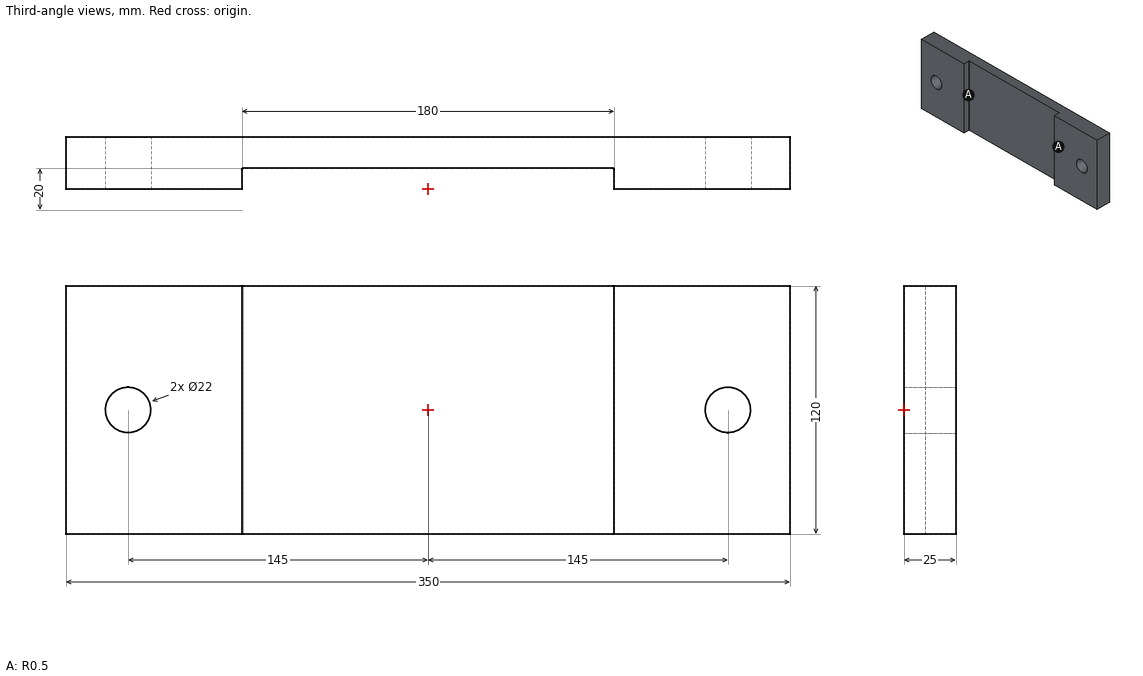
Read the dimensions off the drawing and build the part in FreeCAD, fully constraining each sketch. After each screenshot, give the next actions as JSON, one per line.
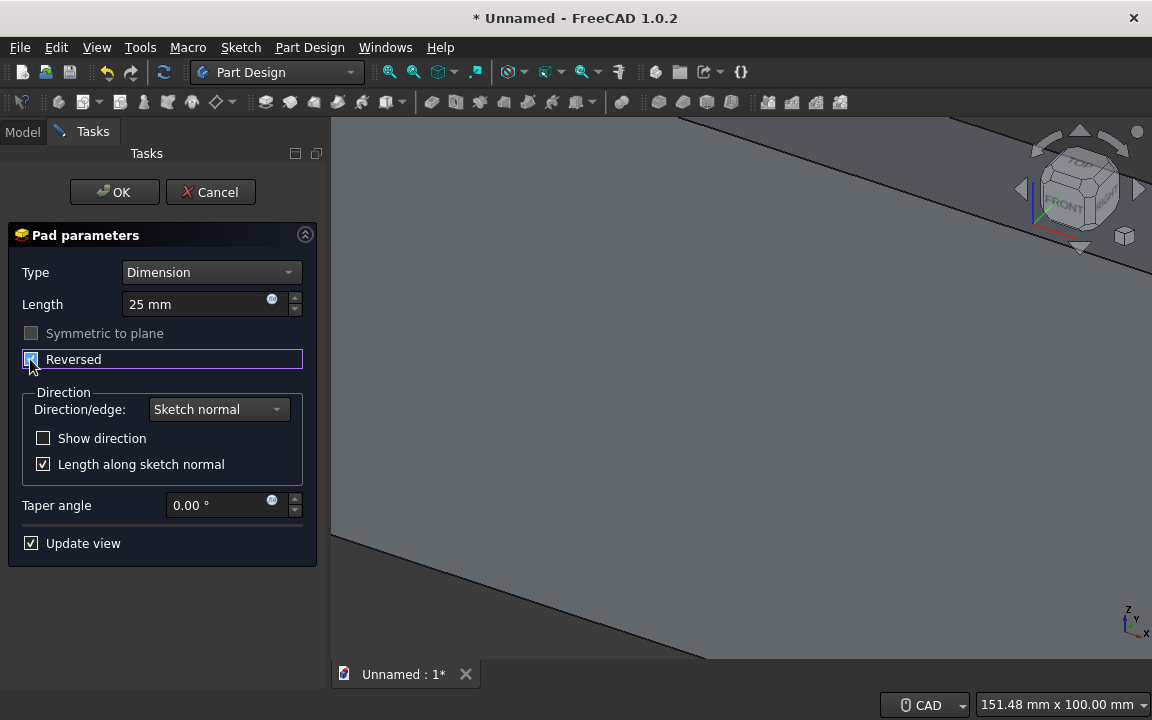
{"action": "left_click", "coordinate": [115, 192]}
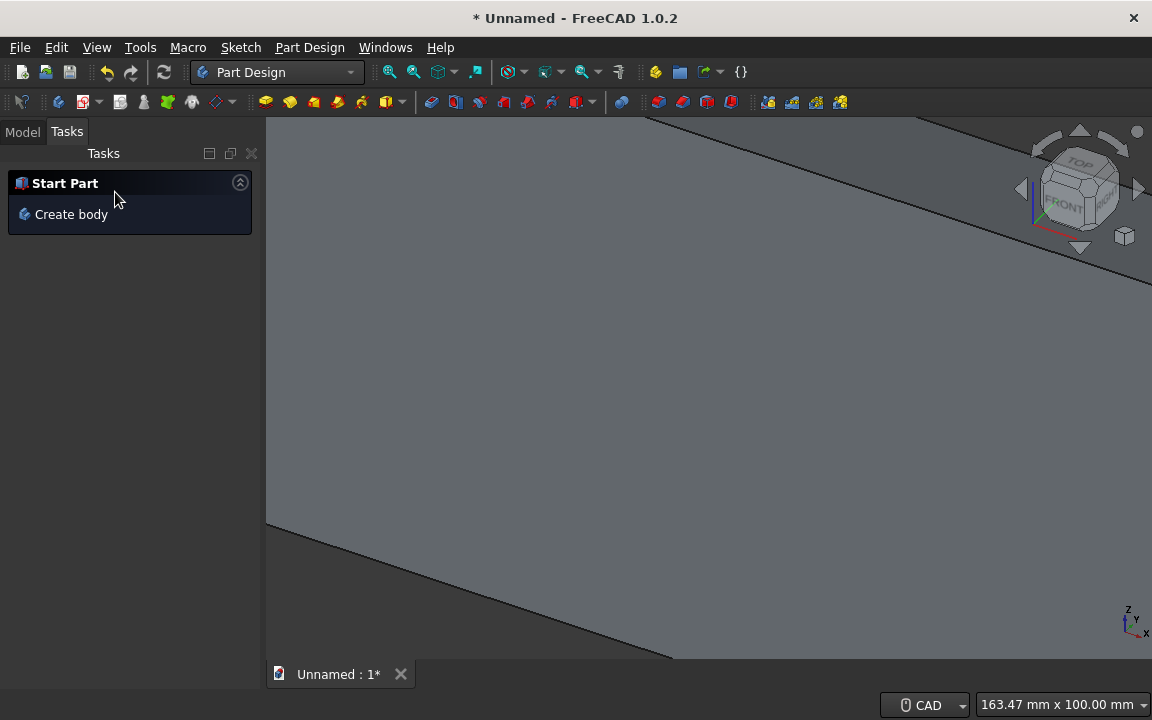
{"action": "left_click", "coordinate": [390, 72]}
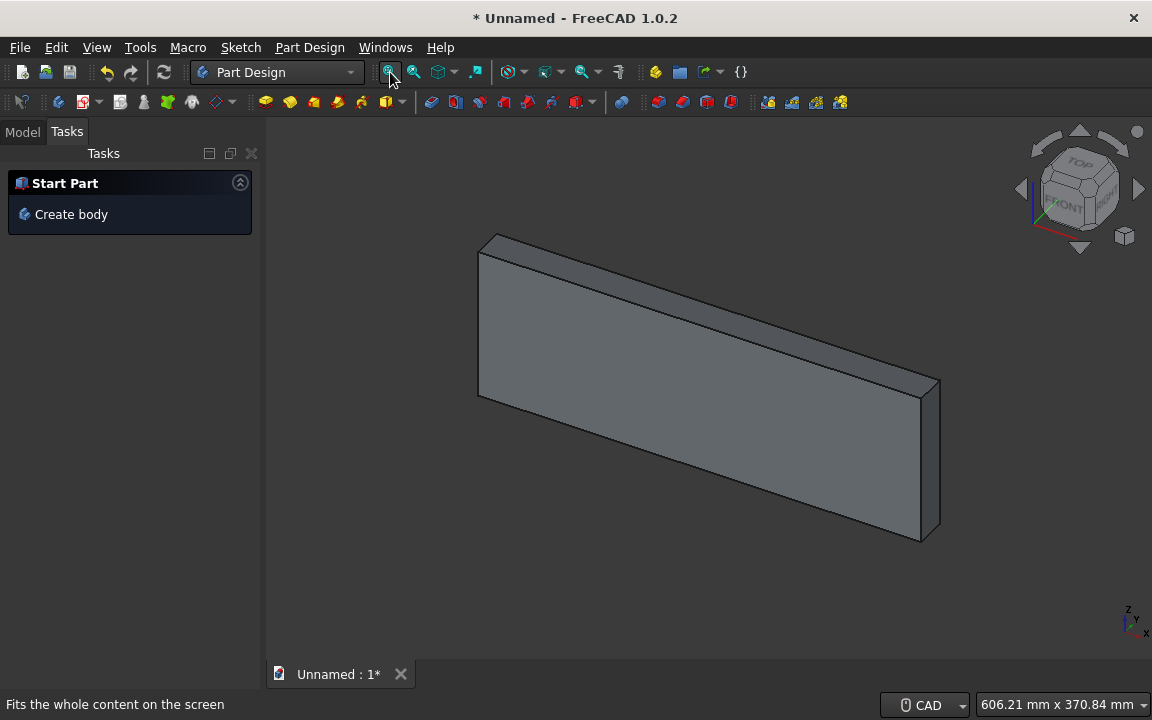
{"action": "left_click", "coordinate": [899, 378]}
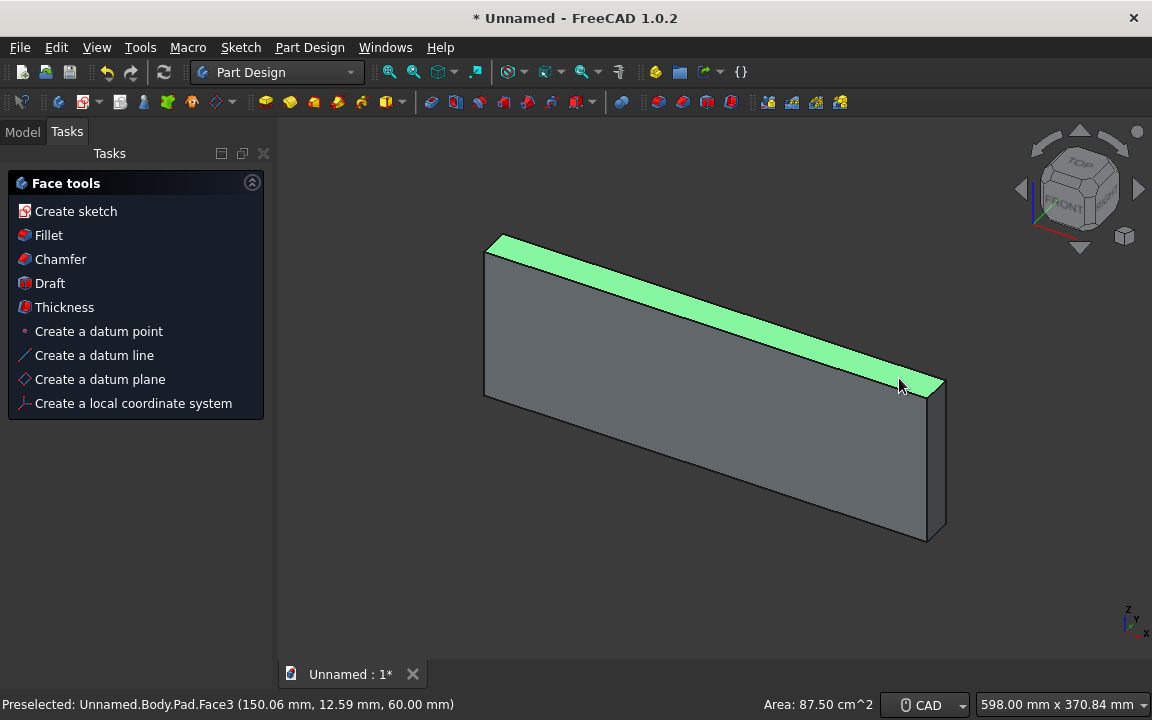
{"action": "left_click", "coordinate": [84, 102]}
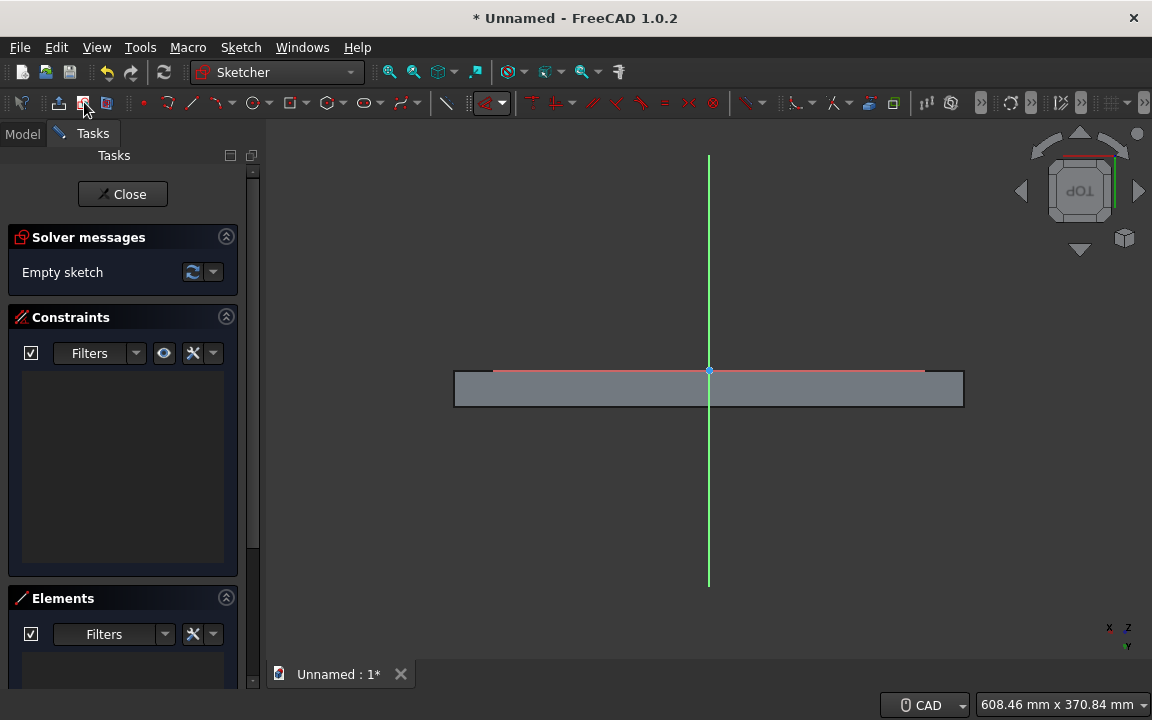
{"action": "scroll", "coordinate": [792, 349], "scroll_direction": "up", "scroll_amount": 3}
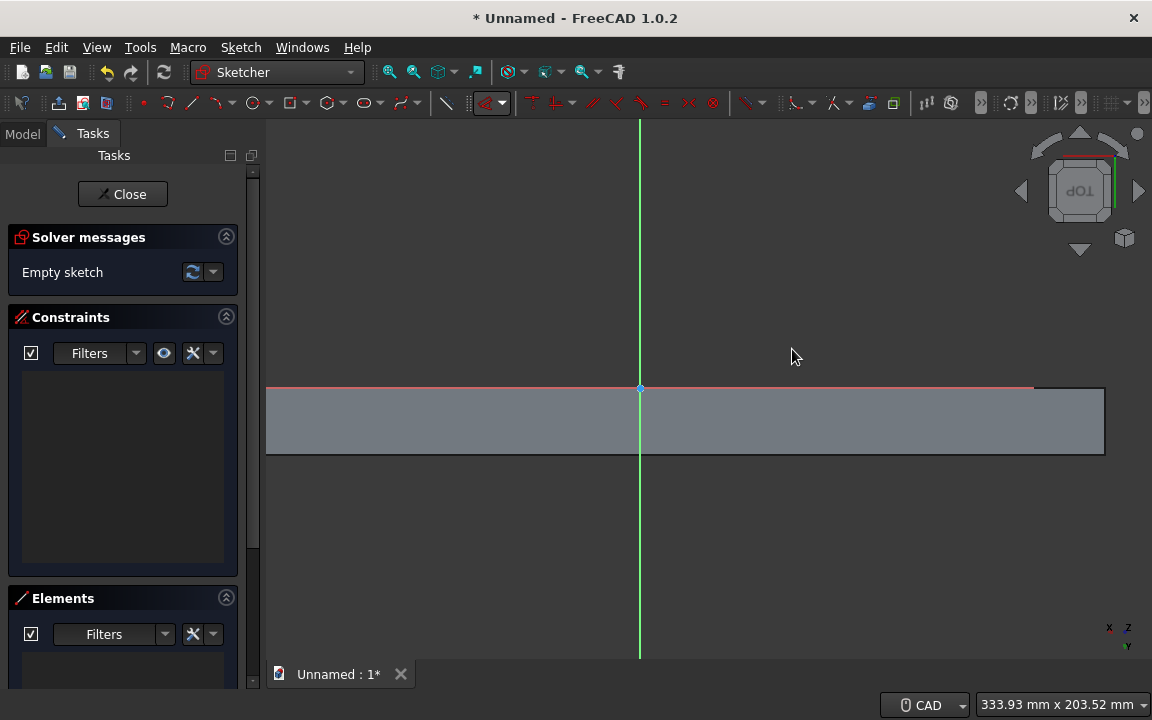
{"action": "left_click", "coordinate": [290, 104]}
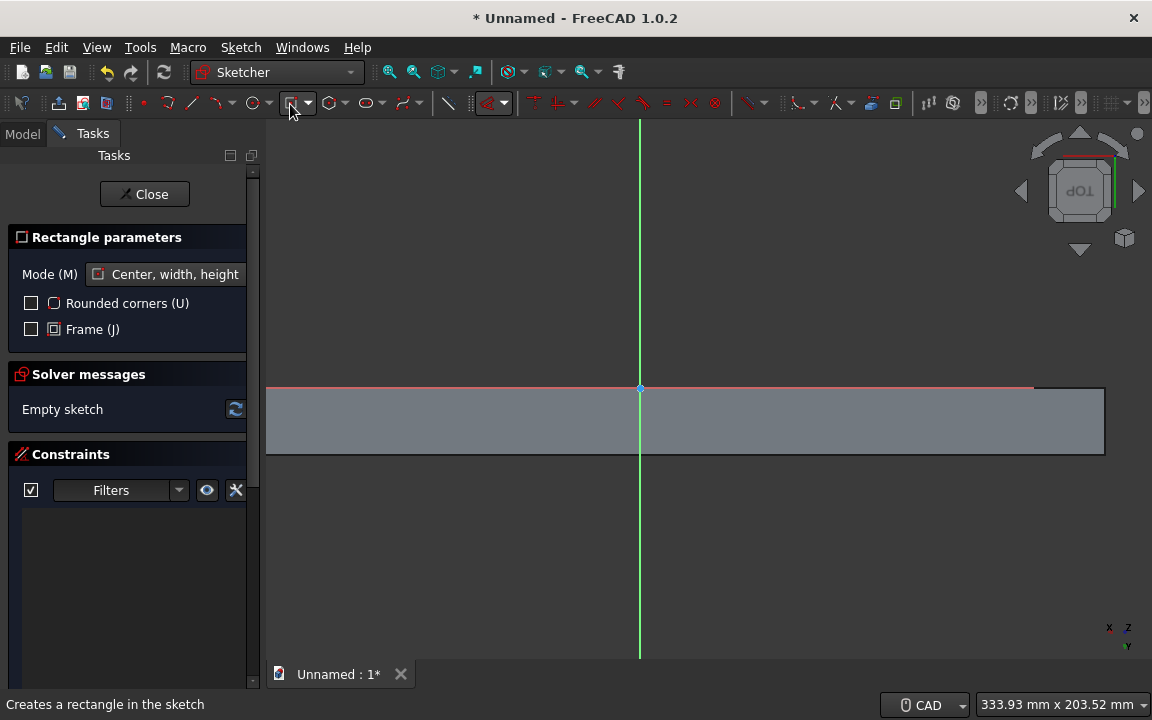
{"action": "left_click", "coordinate": [640, 388]}
{"action": "mouse_move", "coordinate": [879, 362]}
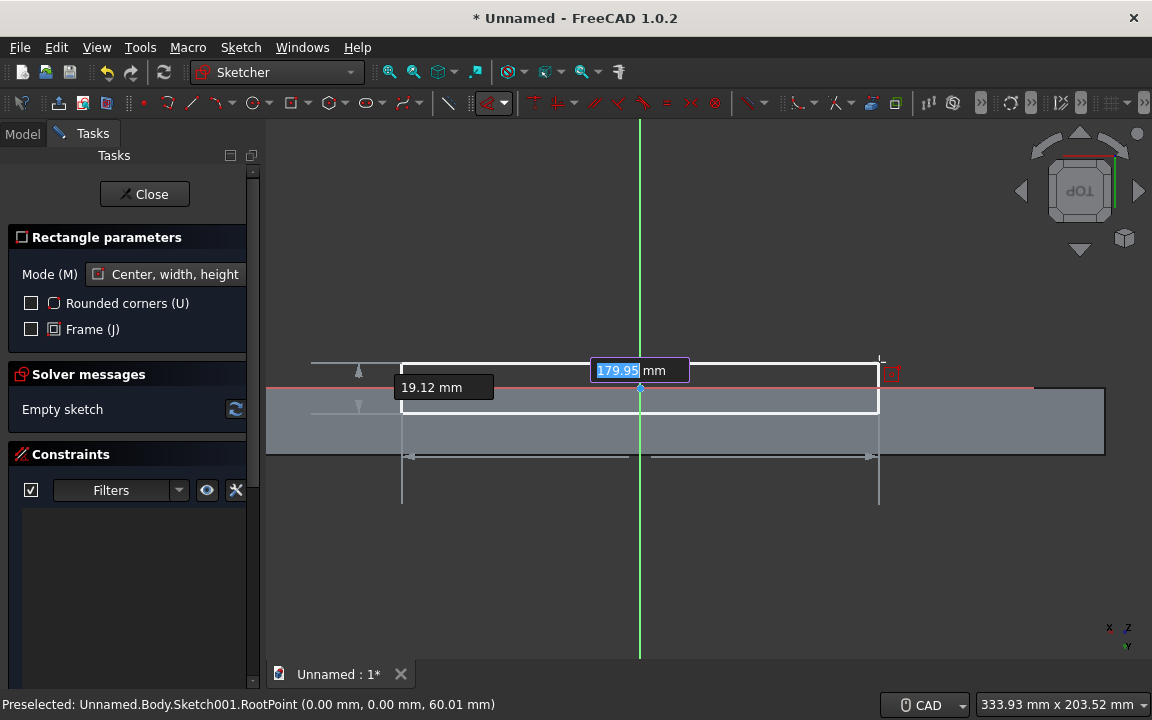
{"action": "type", "text": "180"}
{"action": "key", "text": "Tab"}
{"action": "type", "text": "20"}
{"action": "key", "text": "Return"}
{"action": "key", "text": "Escape"}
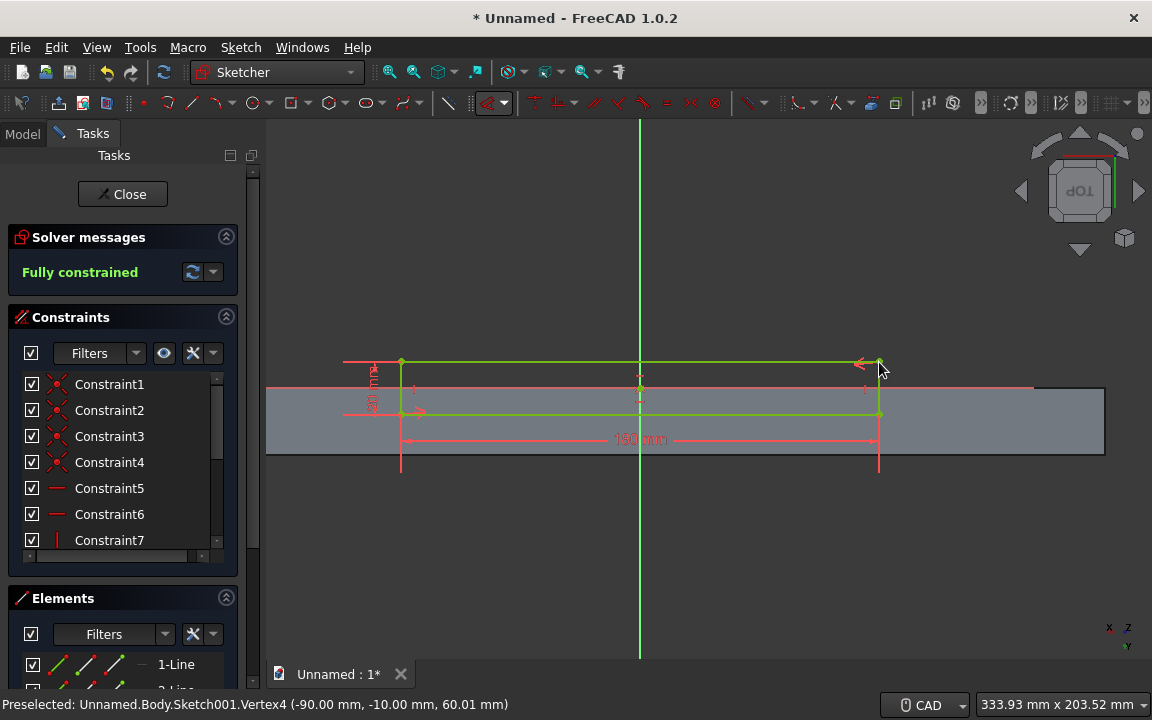
{"action": "left_click", "coordinate": [123, 194]}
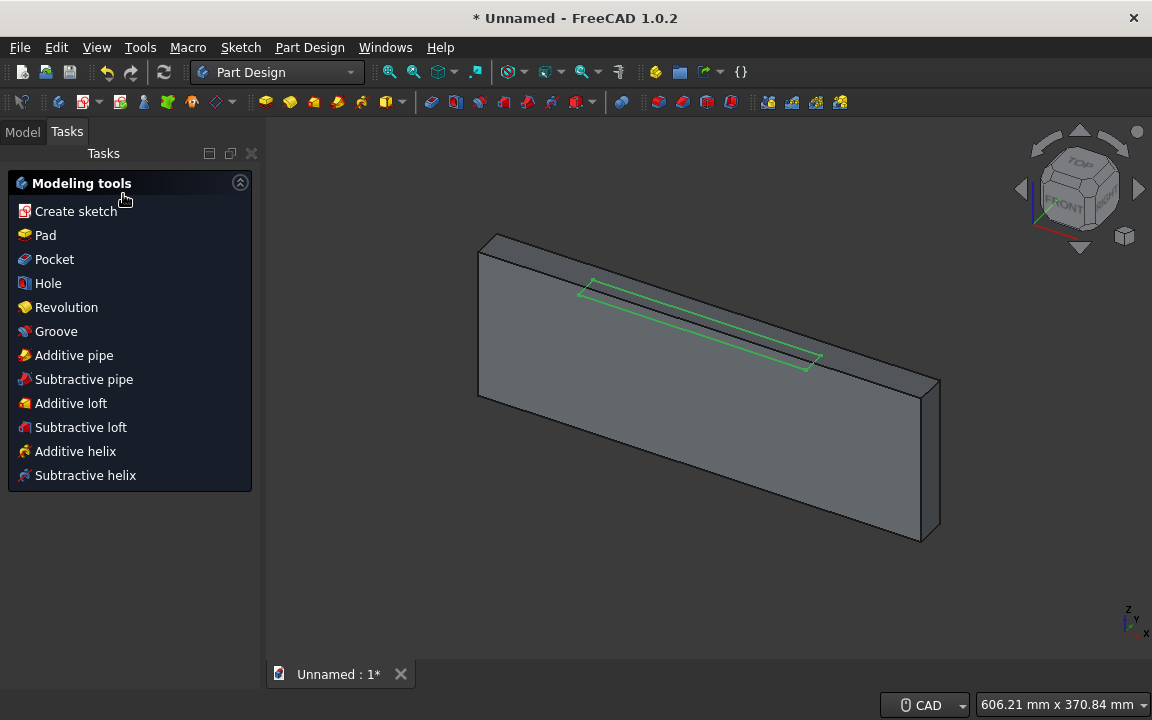
{"action": "left_click", "coordinate": [432, 102]}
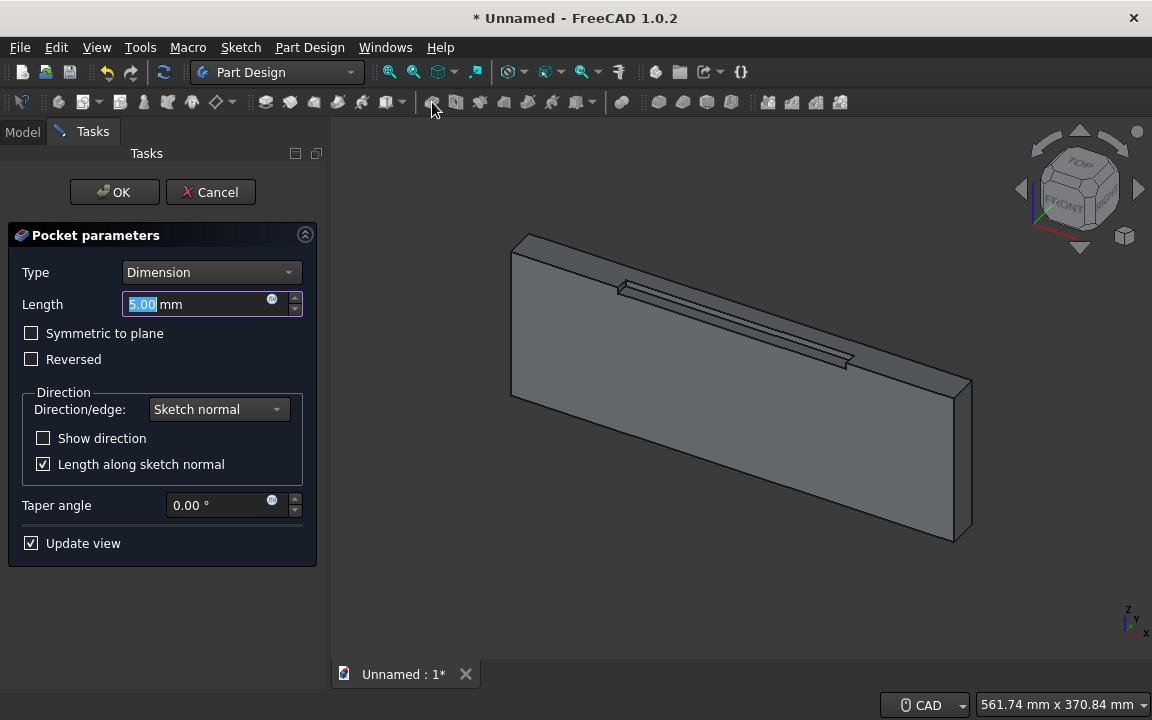
{"action": "left_click", "coordinate": [212, 272]}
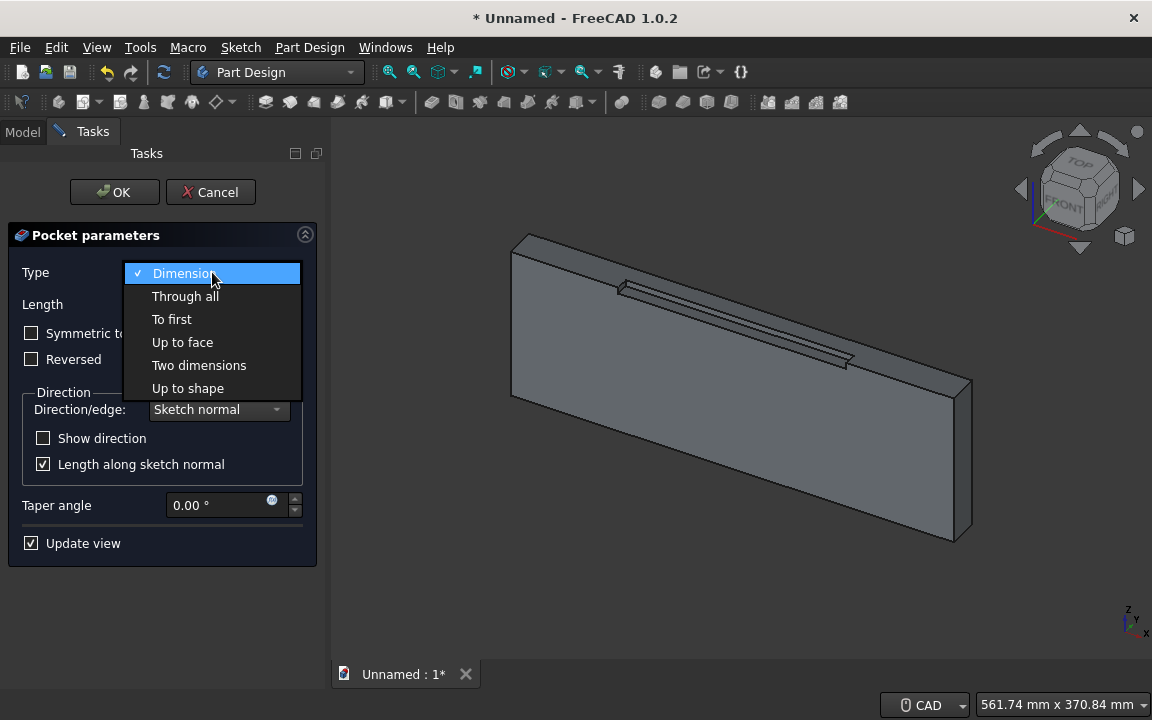
{"action": "left_click", "coordinate": [212, 296]}